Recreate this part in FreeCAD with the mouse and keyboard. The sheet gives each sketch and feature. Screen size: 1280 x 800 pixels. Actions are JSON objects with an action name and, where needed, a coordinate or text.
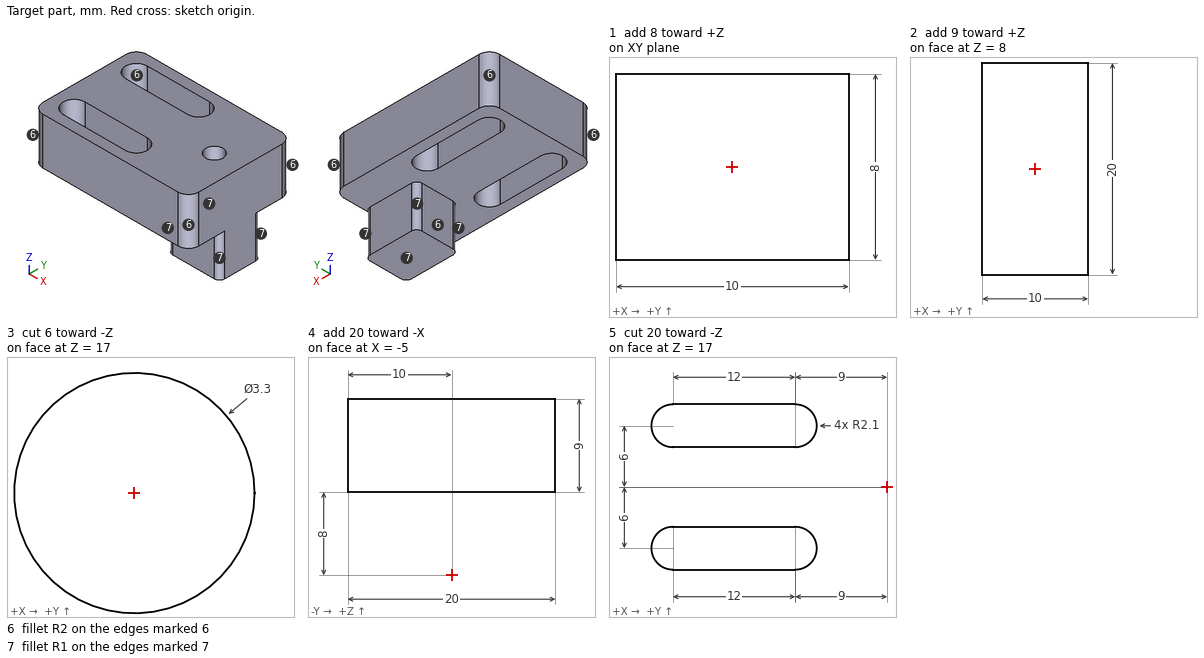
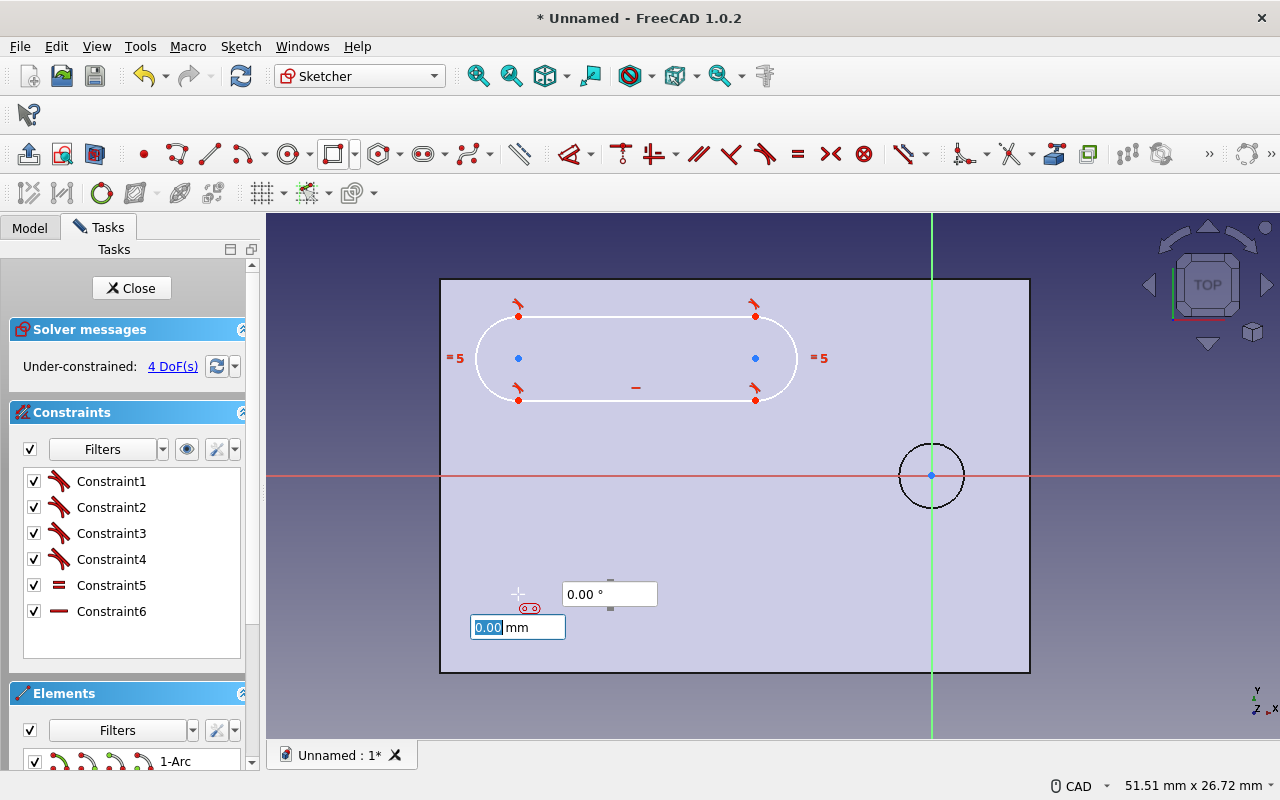
{"action": "left_click", "coordinate": [755, 594]}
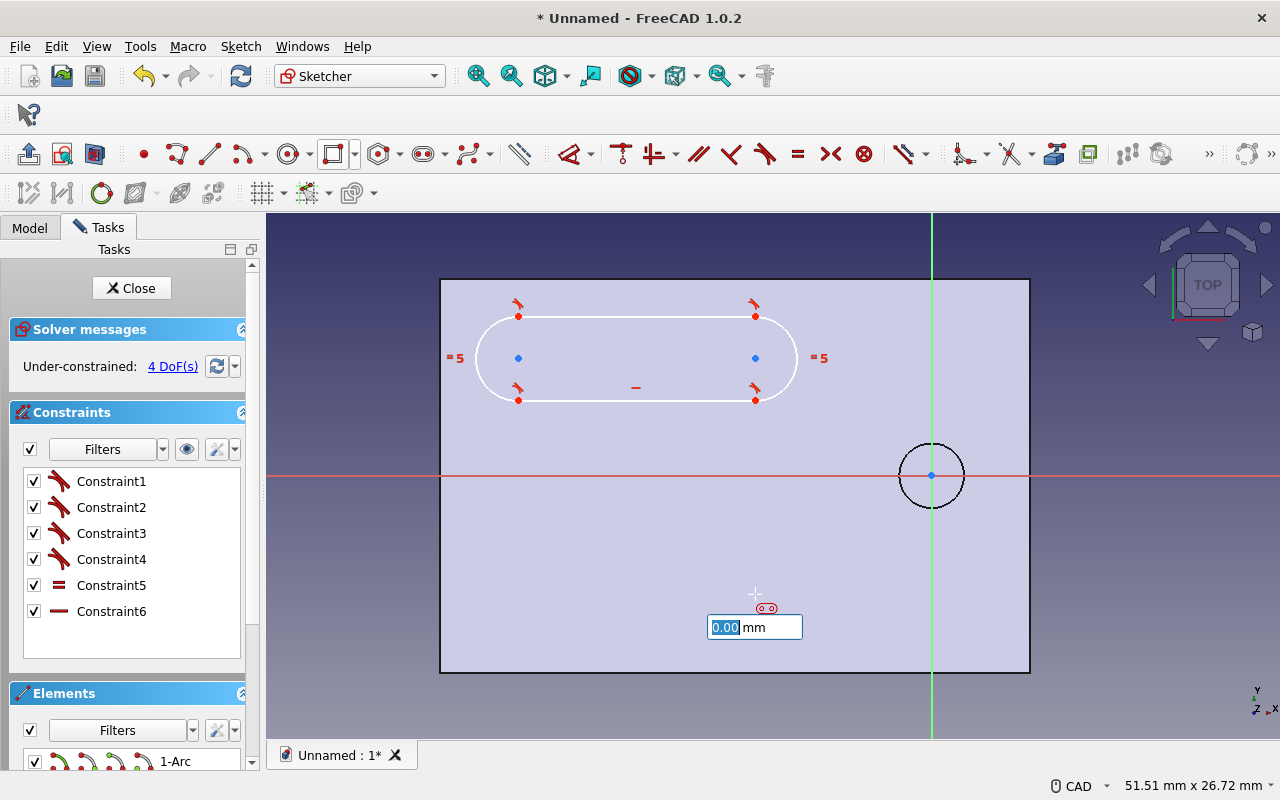
{"action": "left_click", "coordinate": [636, 635]}
{"action": "key", "text": "Escape"}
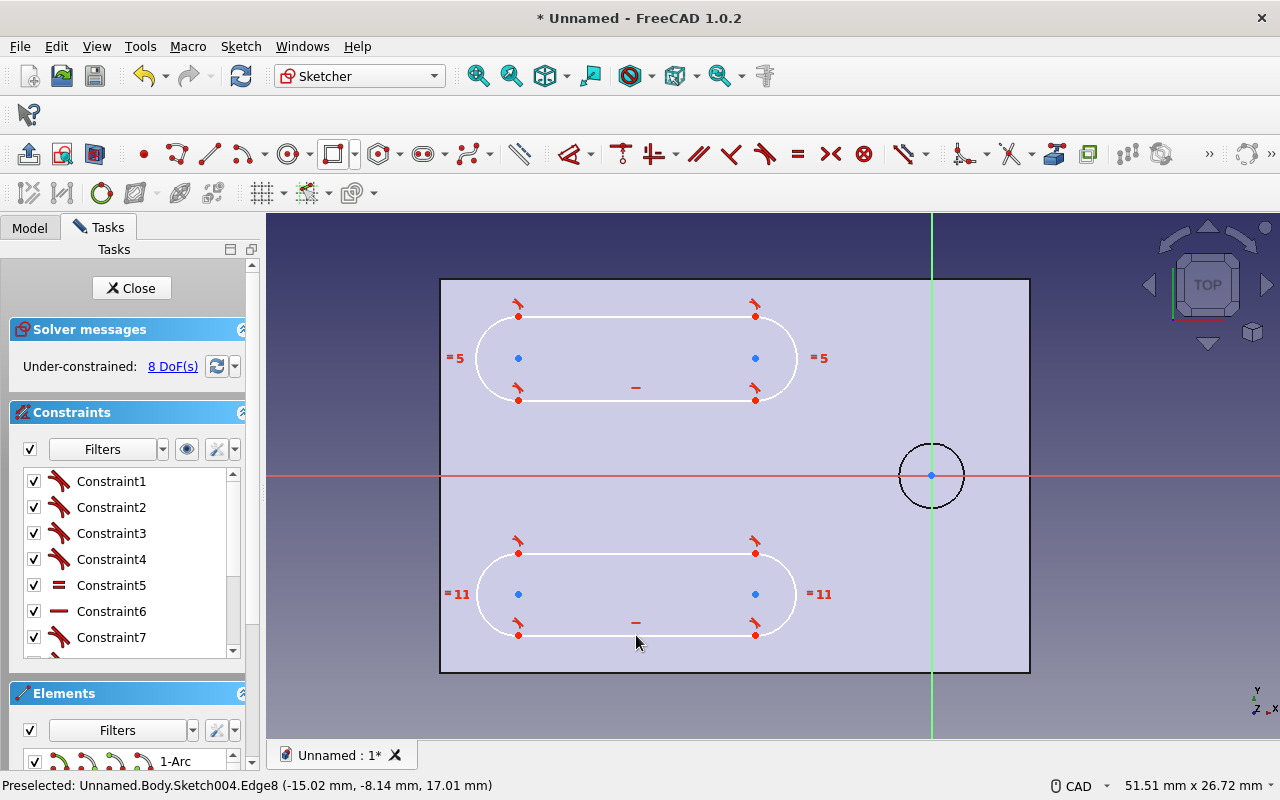
{"action": "left_click", "coordinate": [484, 334]}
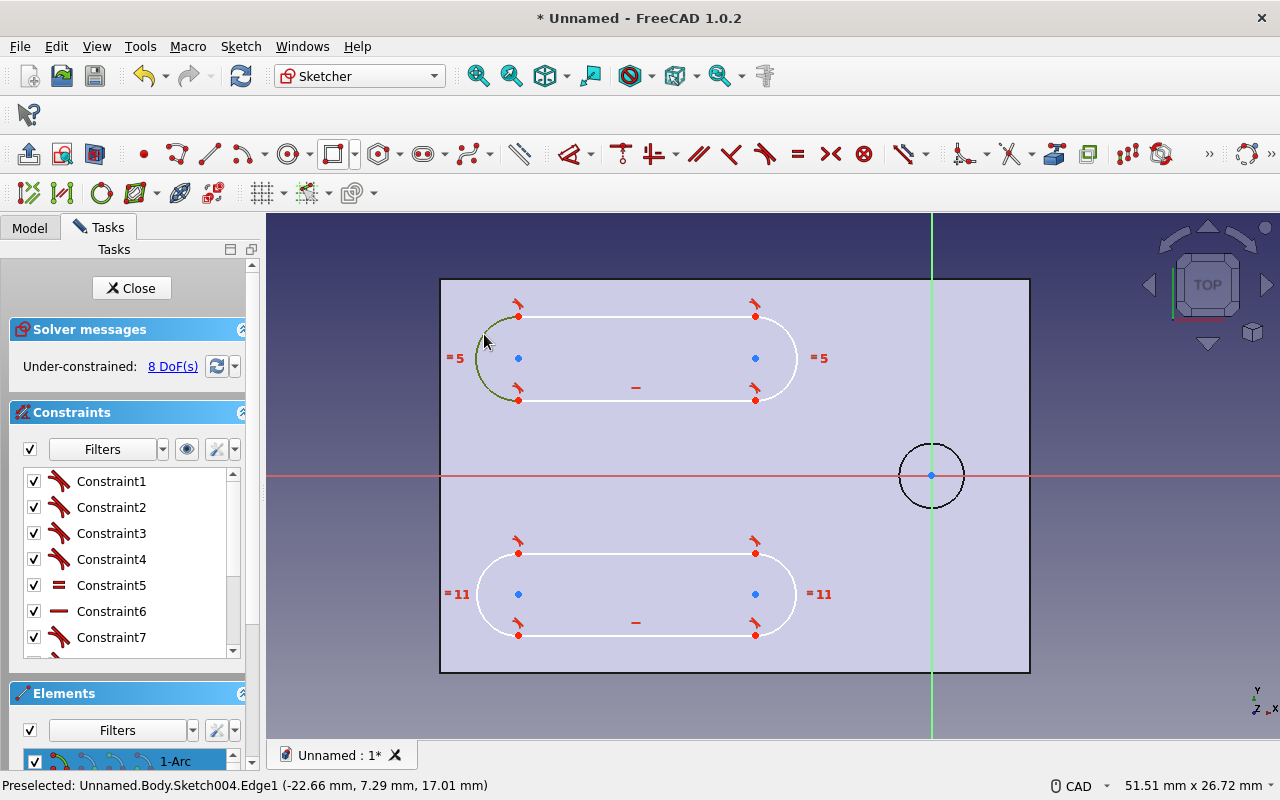
{"action": "left_click", "coordinate": [485, 571]}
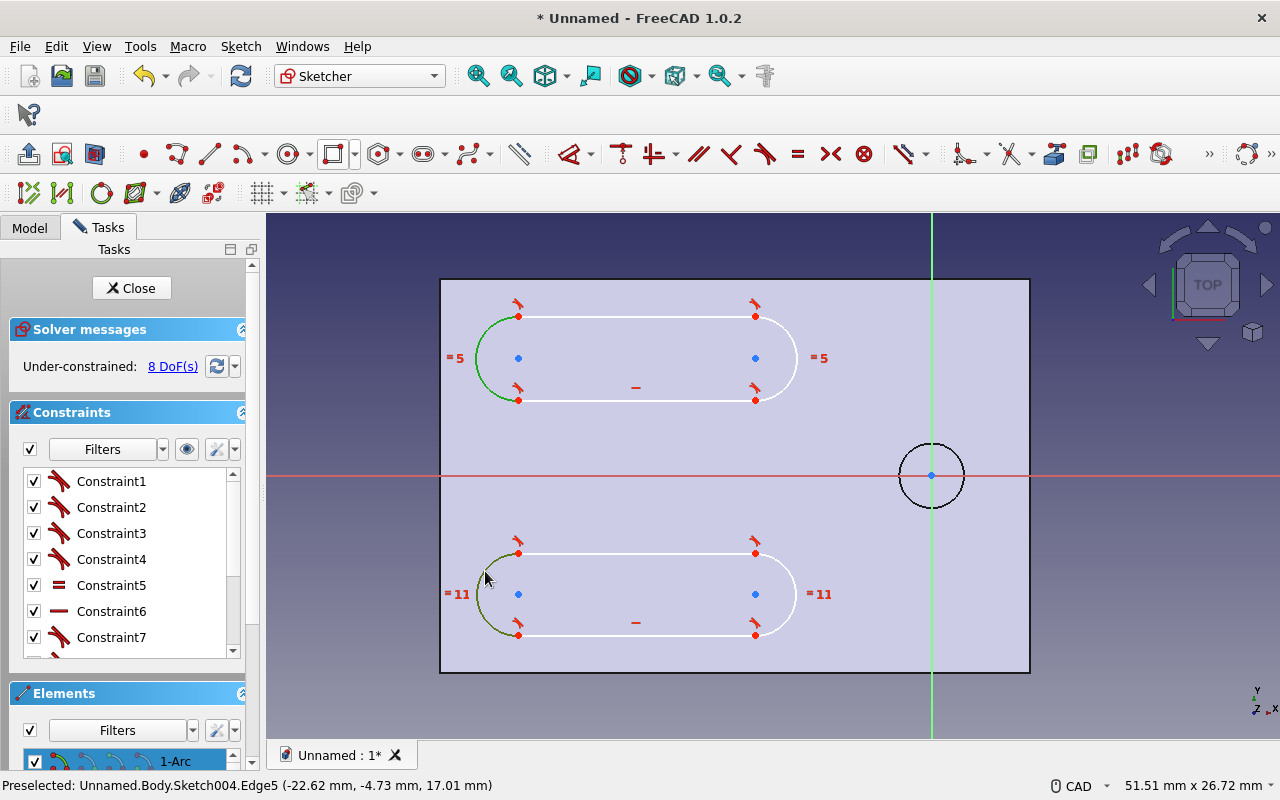
{"action": "key", "text": "e"}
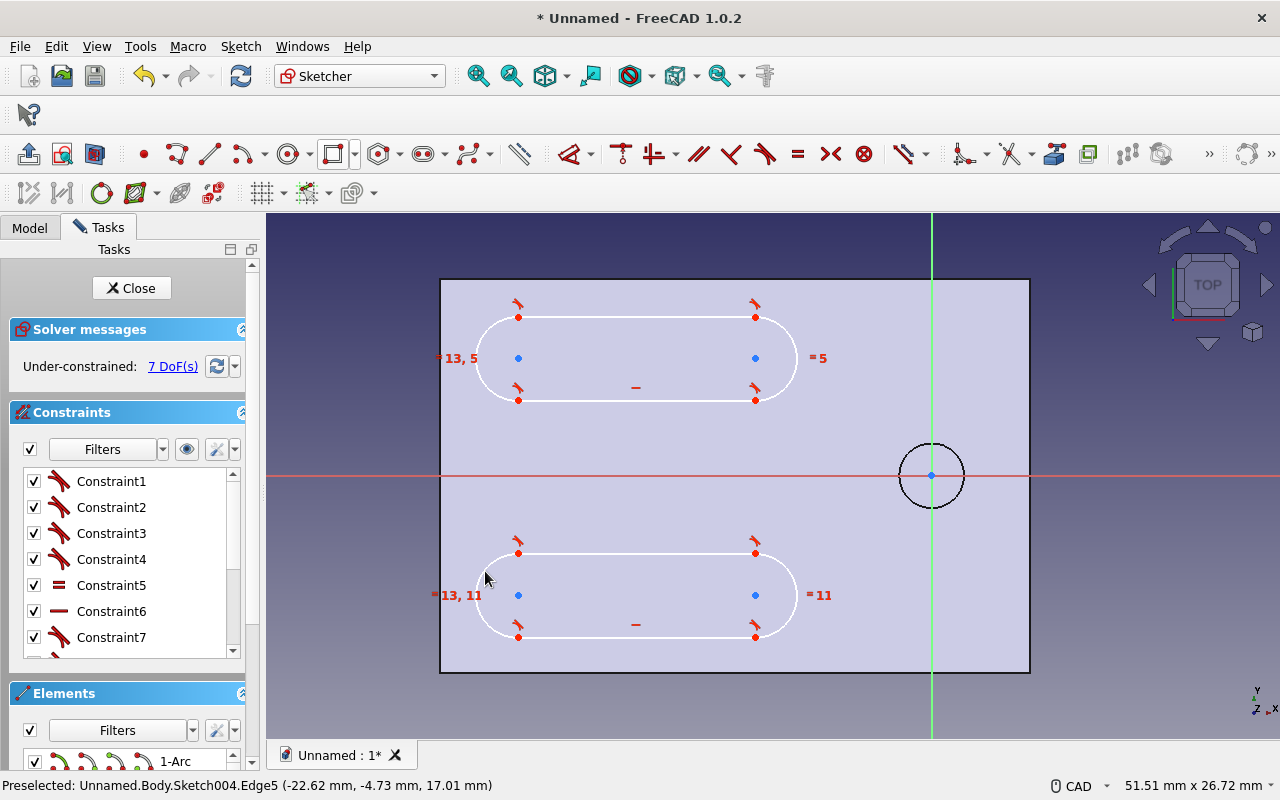
{"action": "left_click", "coordinate": [568, 154]}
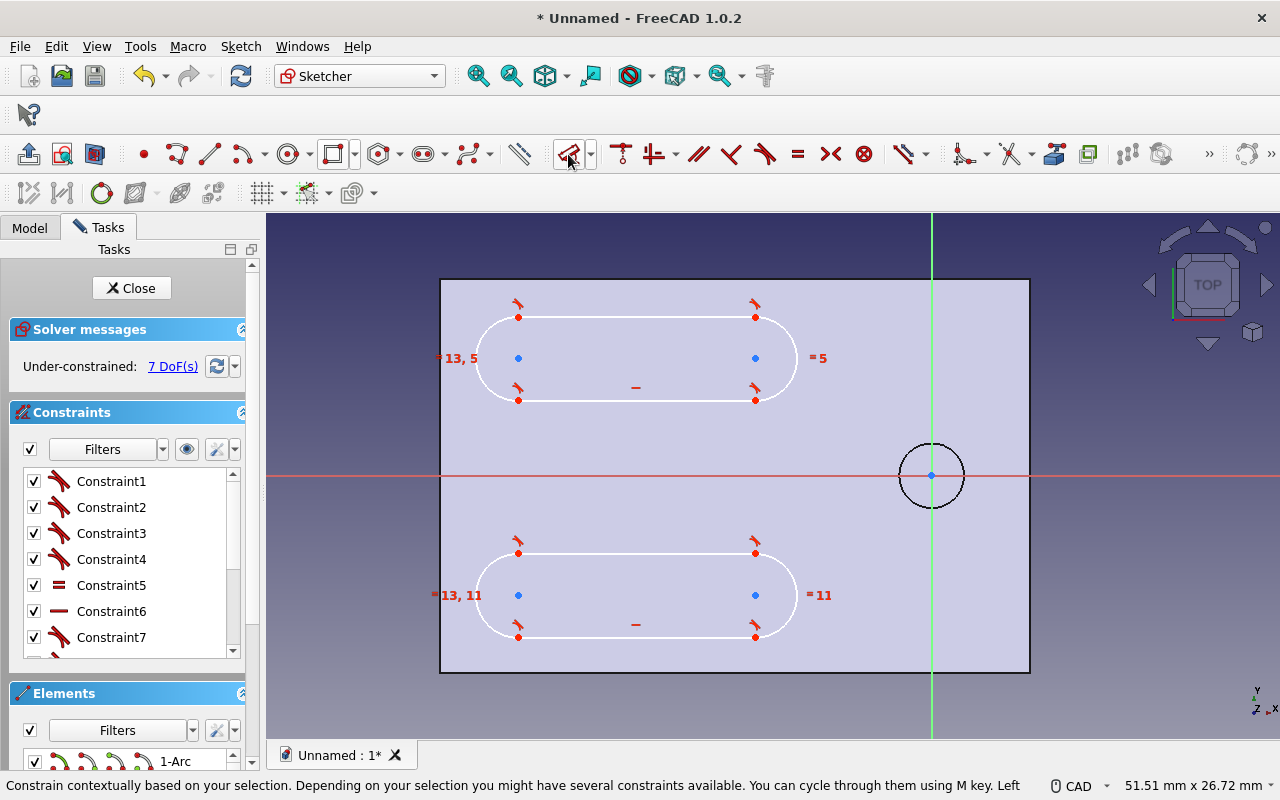
{"action": "left_click", "coordinate": [484, 334]}
{"action": "left_click", "coordinate": [458, 315]}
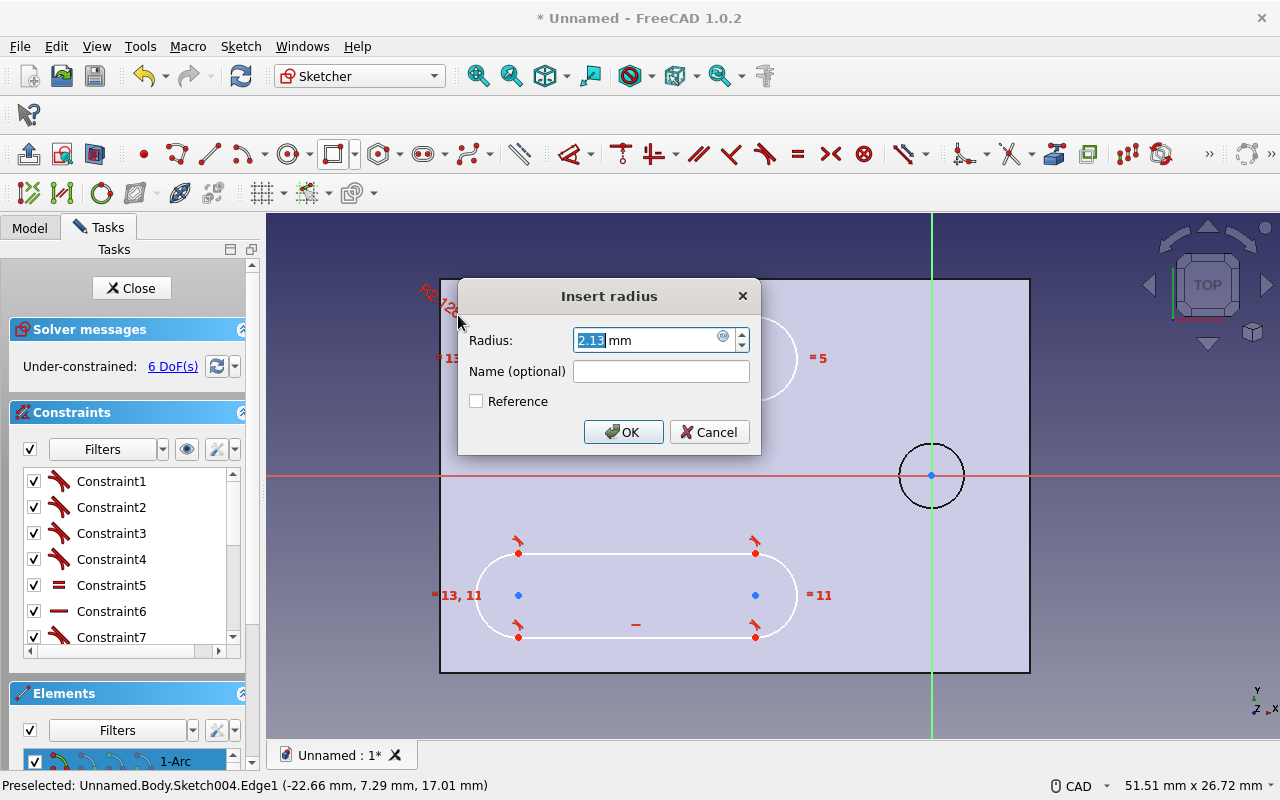
{"action": "type", "text": "2.1"}
{"action": "key", "text": "Return"}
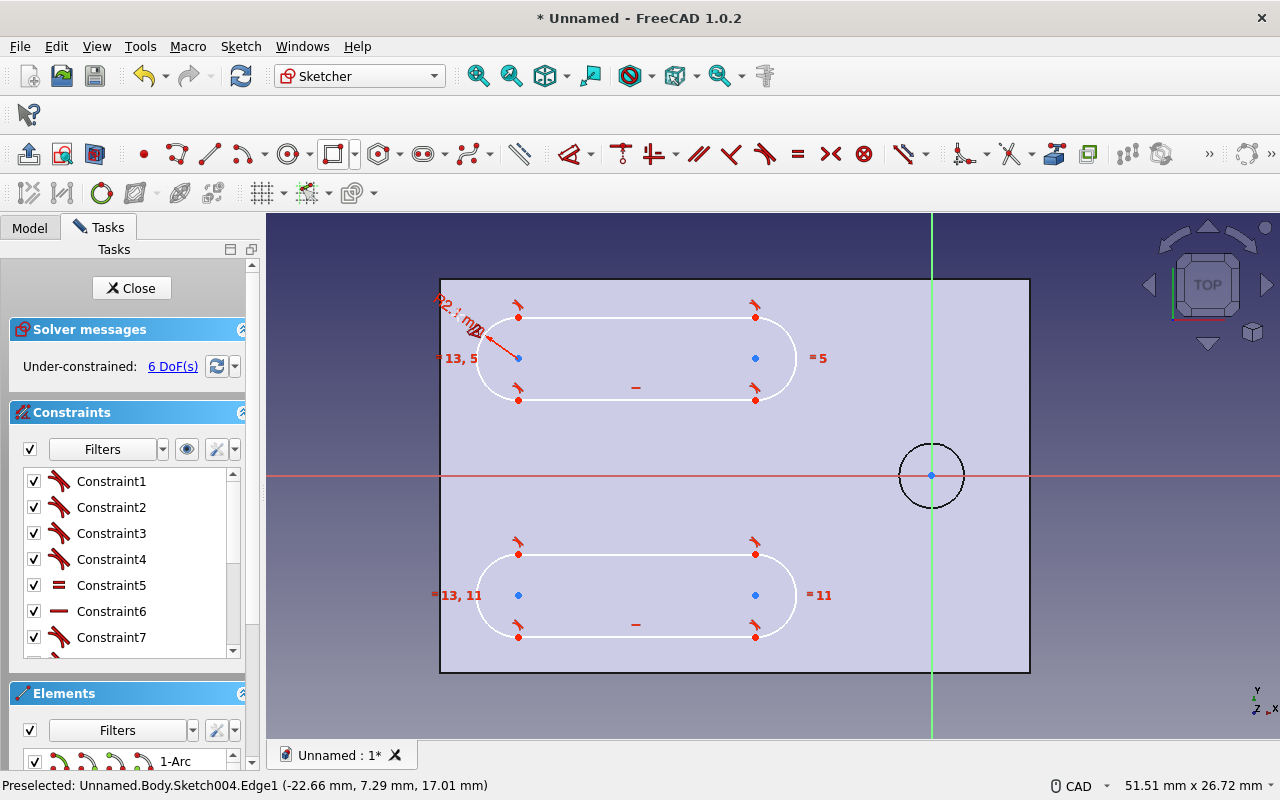
{"action": "left_click", "coordinate": [589, 318]}
{"action": "left_click", "coordinate": [637, 284]}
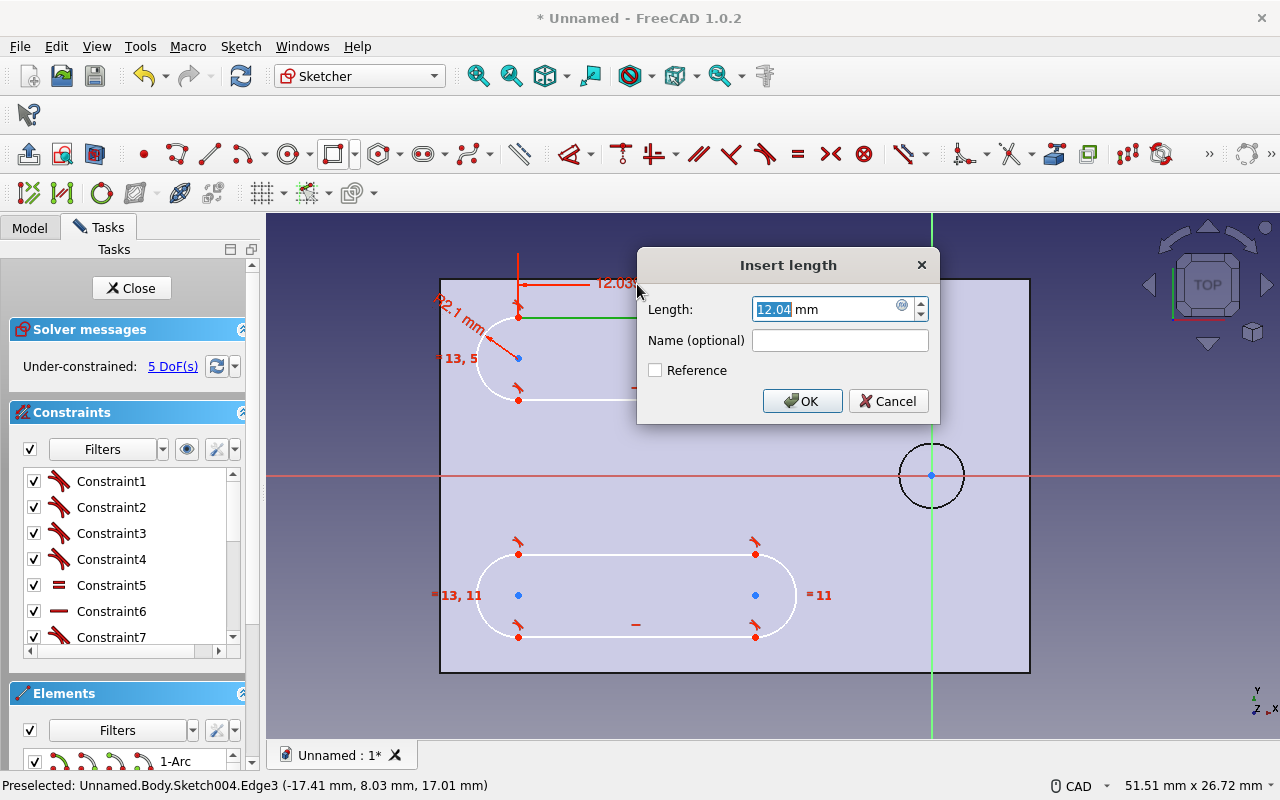
{"action": "type", "text": "12"}
{"action": "key", "text": "Return"}